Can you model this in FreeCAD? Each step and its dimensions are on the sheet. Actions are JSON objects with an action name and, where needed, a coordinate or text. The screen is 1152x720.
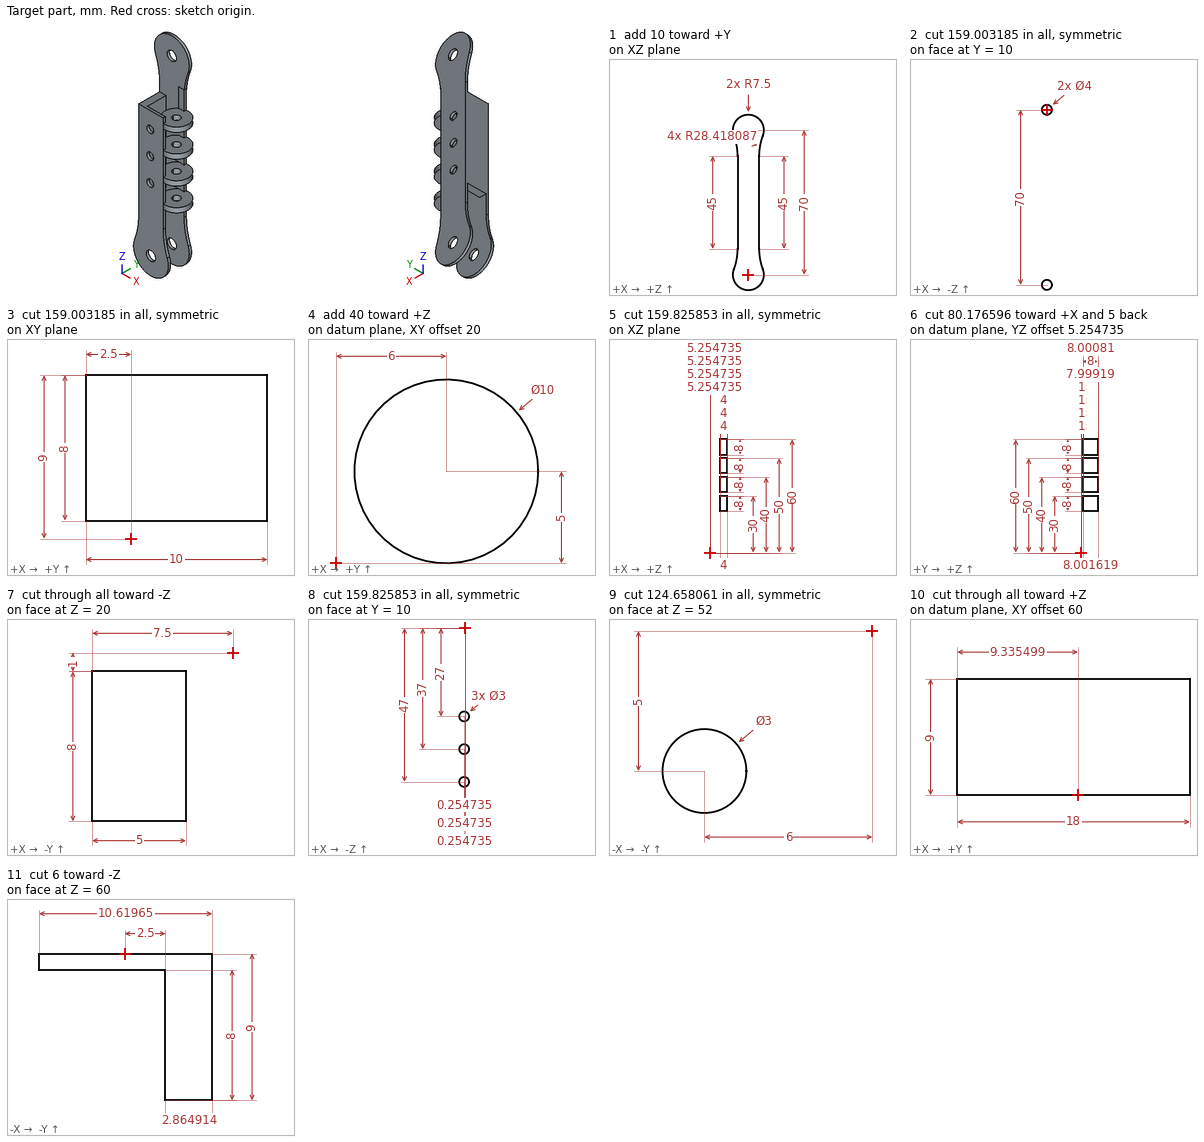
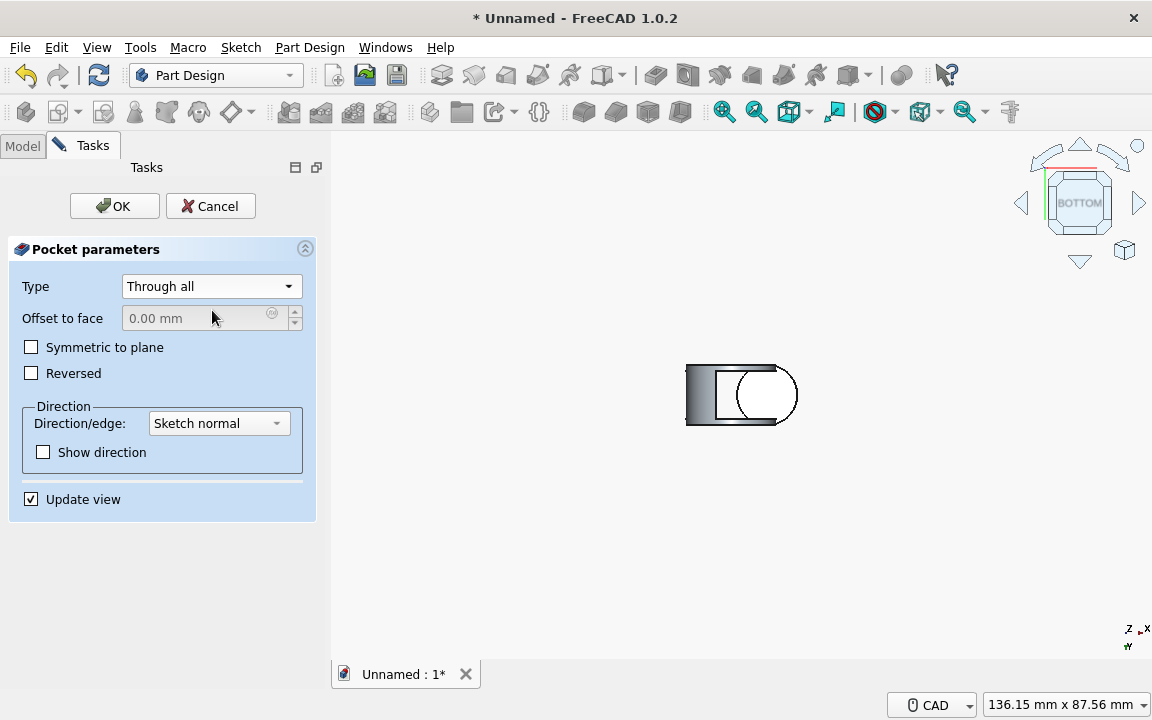
{"action": "left_click", "coordinate": [30, 373]}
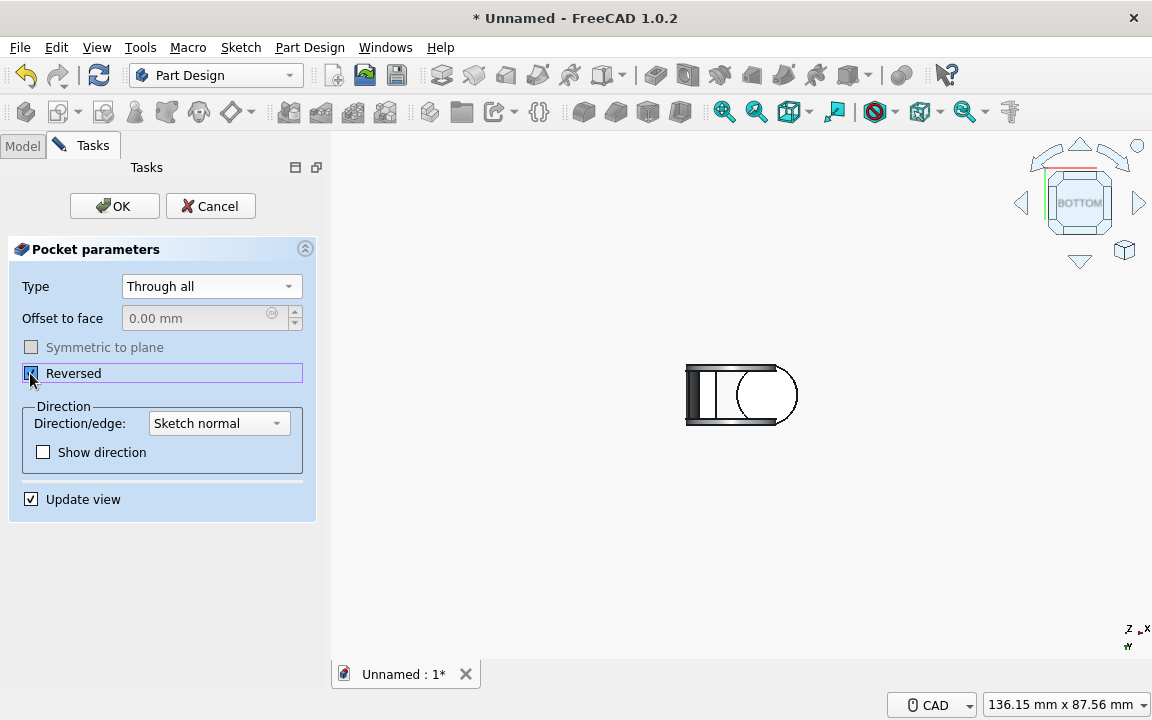
{"action": "left_click", "coordinate": [115, 206]}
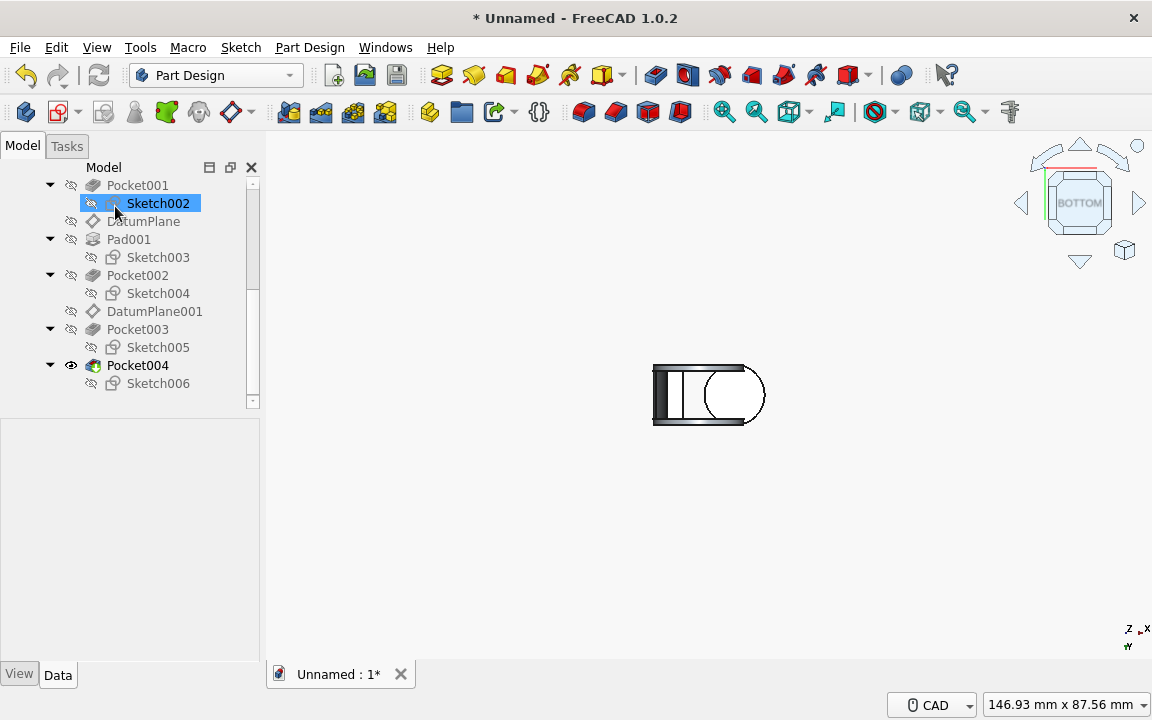
{"action": "left_click", "coordinate": [726, 112]}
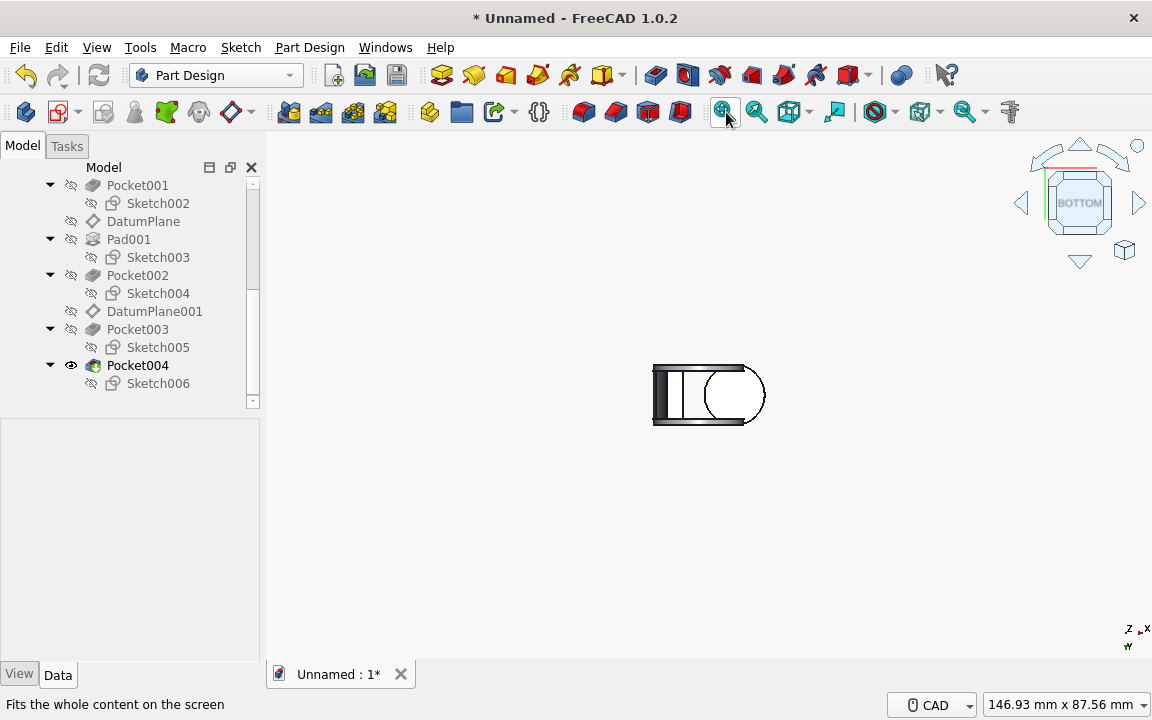
{"action": "key", "text": "4"}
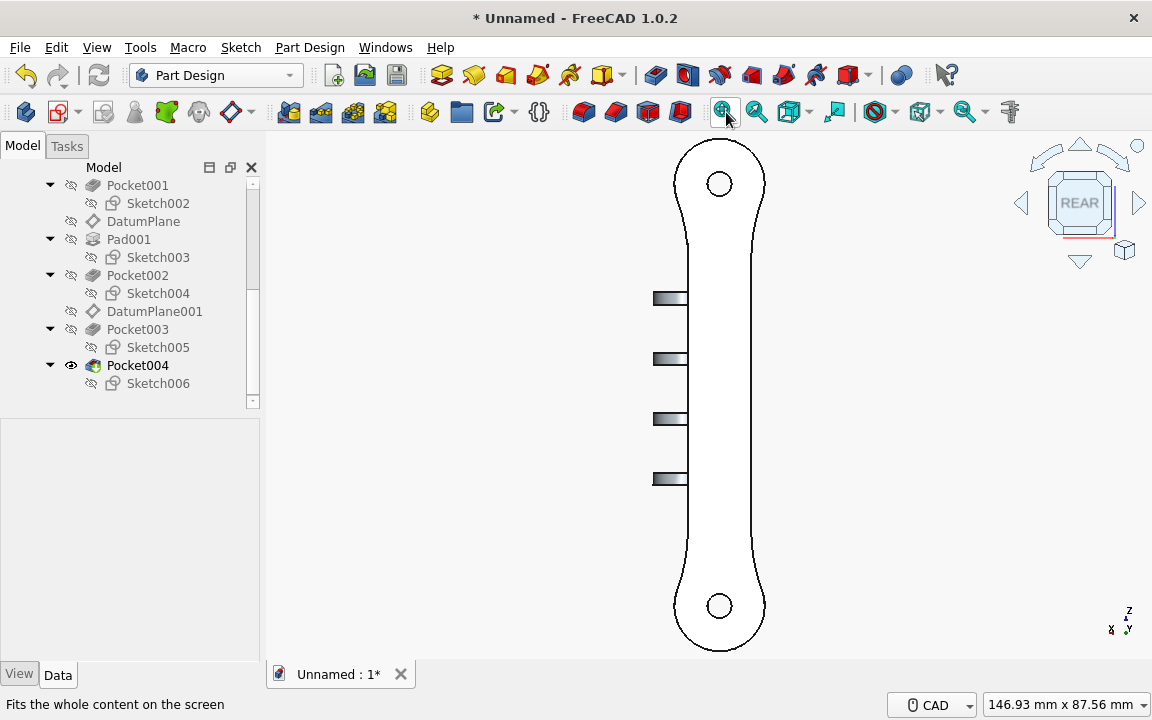
{"action": "left_click", "coordinate": [720, 540]}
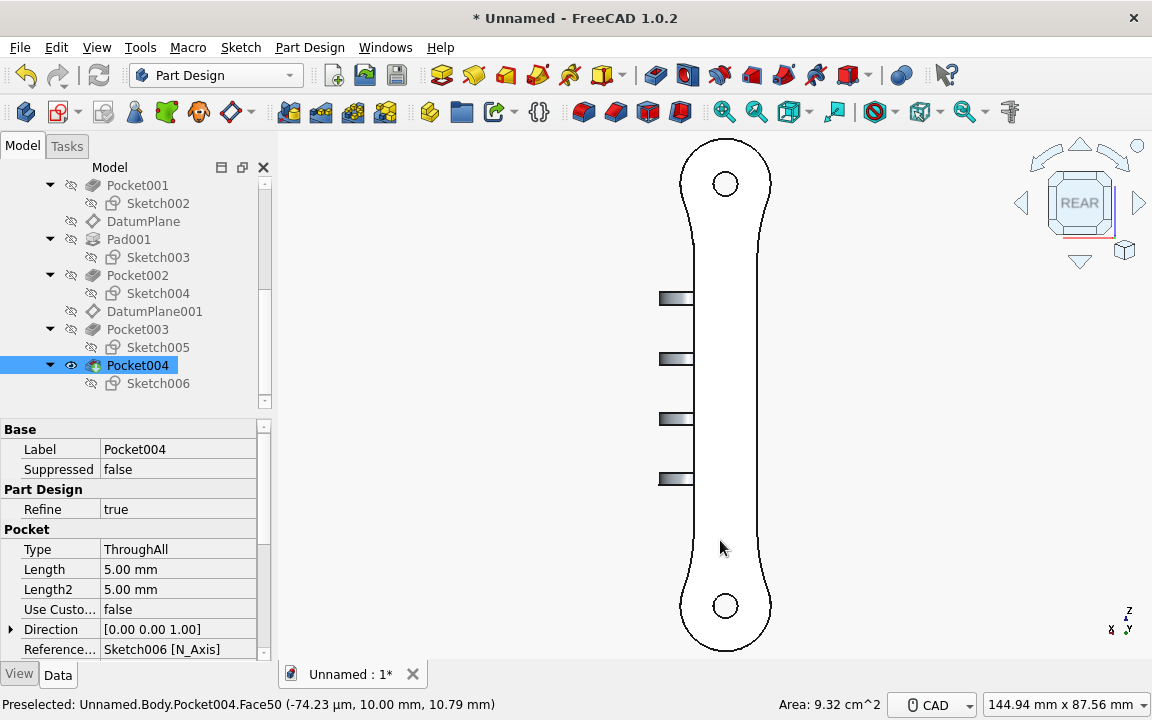
{"action": "left_click", "coordinate": [58, 112]}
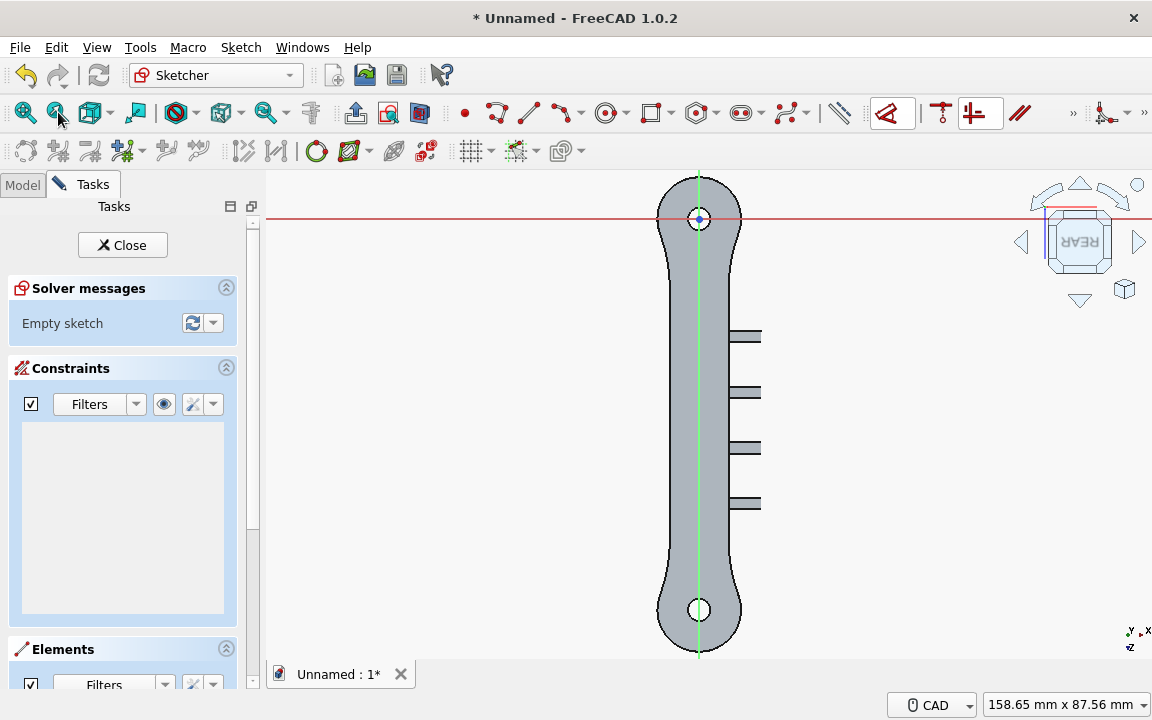
{"action": "scroll", "coordinate": [957, 198], "scroll_direction": "up", "scroll_amount": 1}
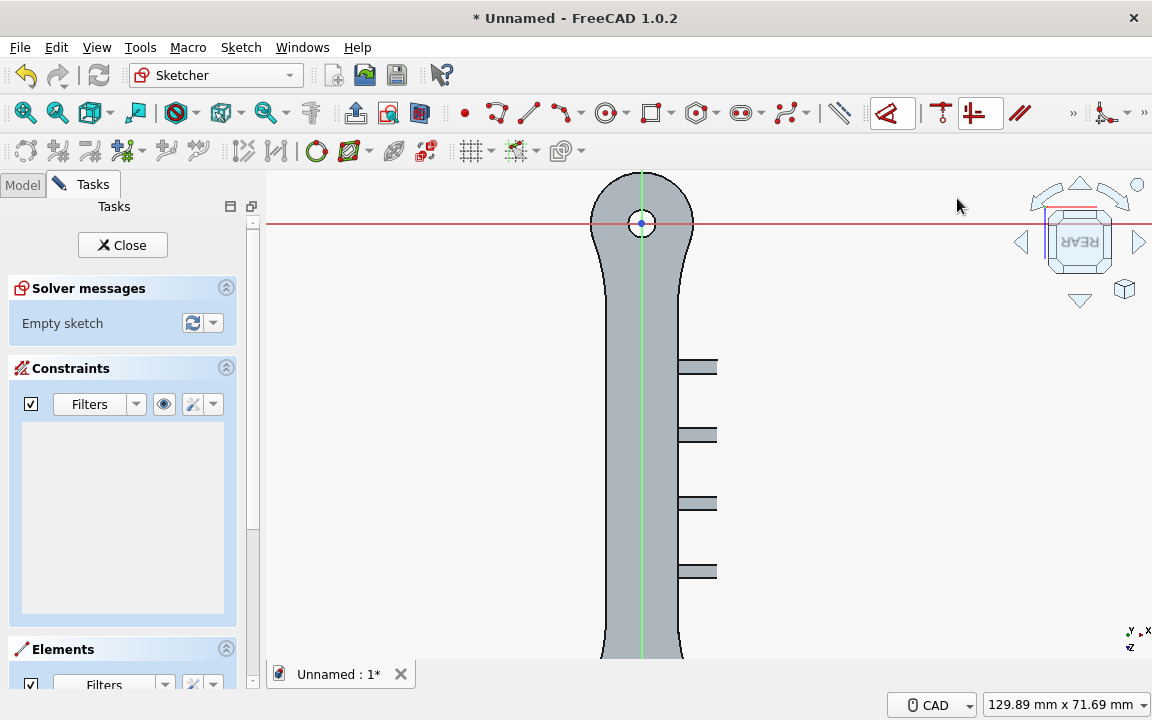
{"action": "key", "text": "g c"}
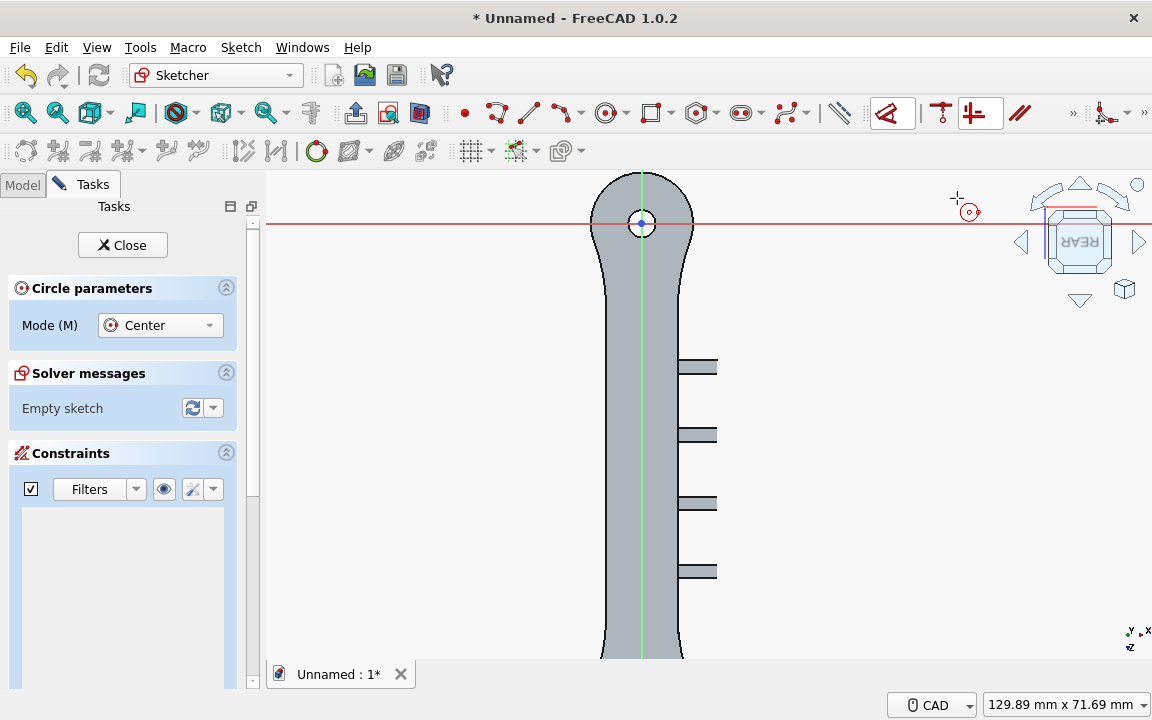
{"action": "scroll", "coordinate": [640, 408], "scroll_direction": "up", "scroll_amount": 12}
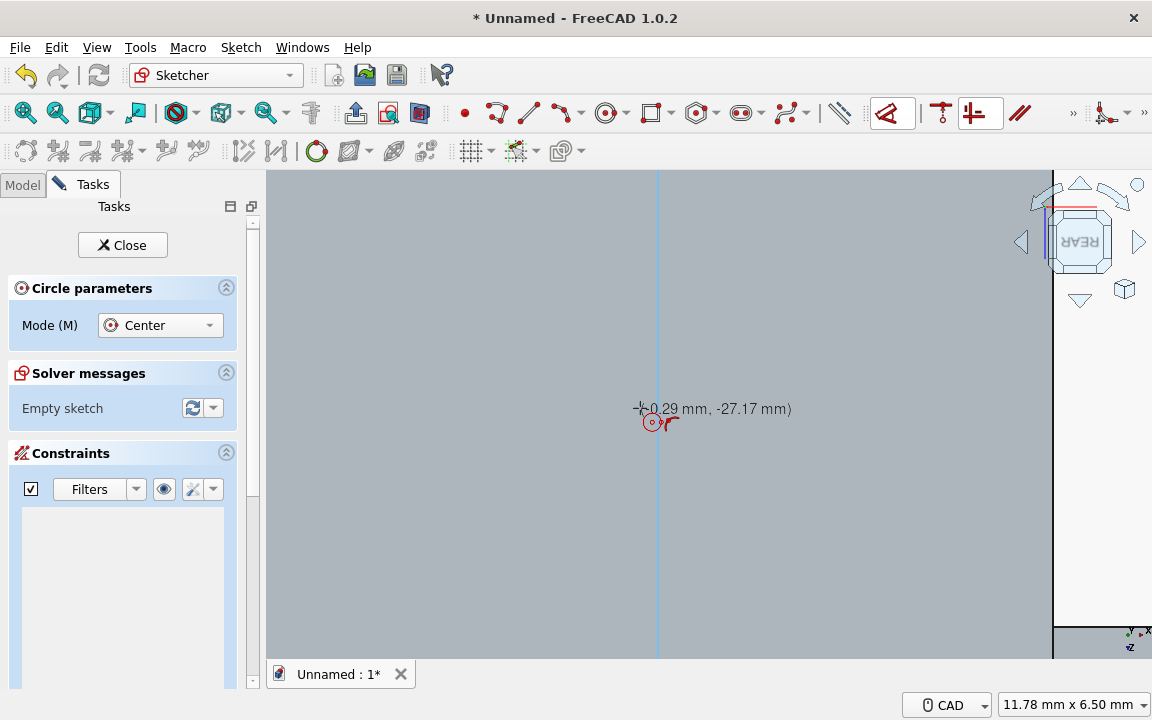
{"action": "left_click", "coordinate": [638, 401]}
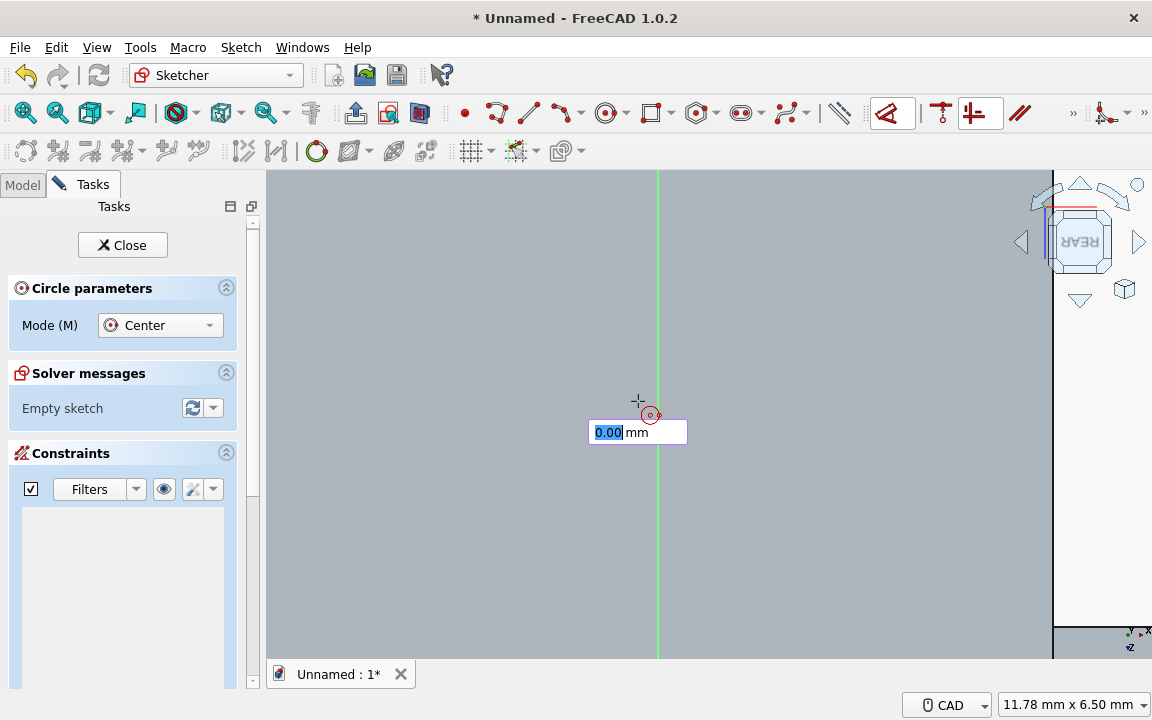
{"action": "scroll", "coordinate": [641, 436], "scroll_direction": "down", "scroll_amount": 12}